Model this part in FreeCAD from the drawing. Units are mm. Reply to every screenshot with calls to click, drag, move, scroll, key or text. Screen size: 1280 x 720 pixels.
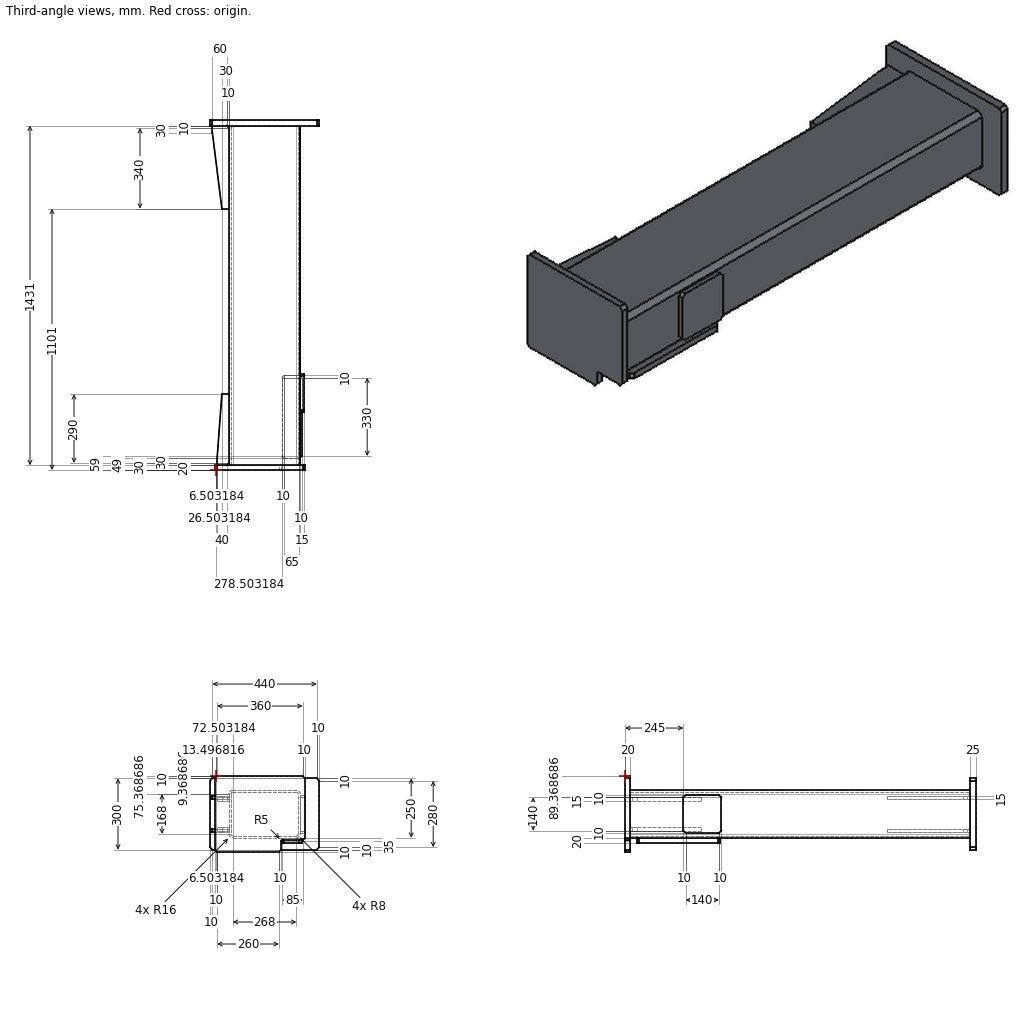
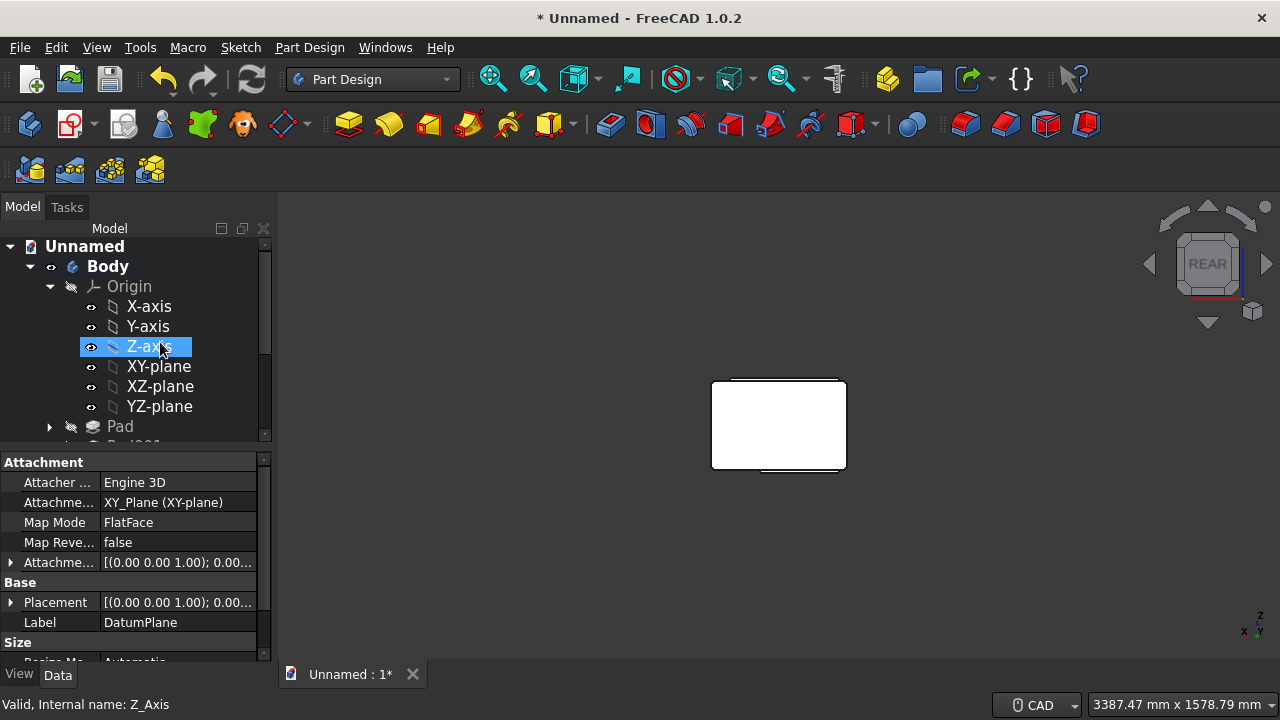
click(136, 367)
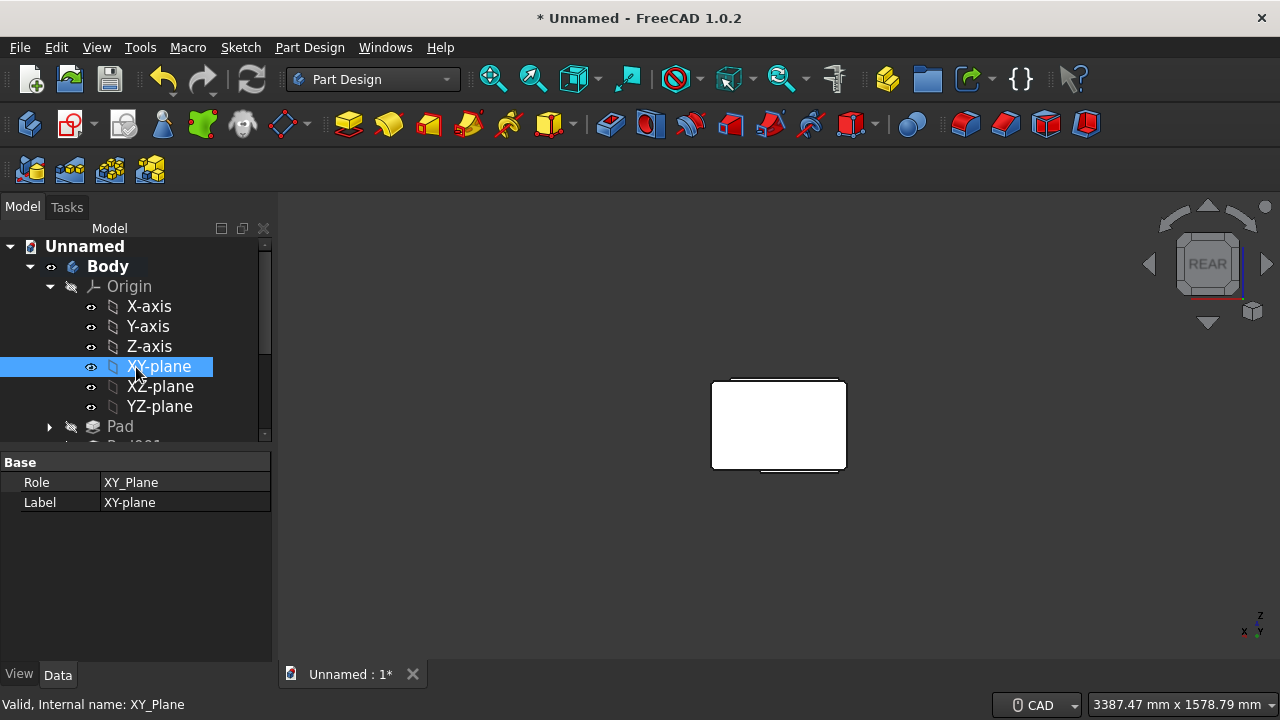
click(284, 124)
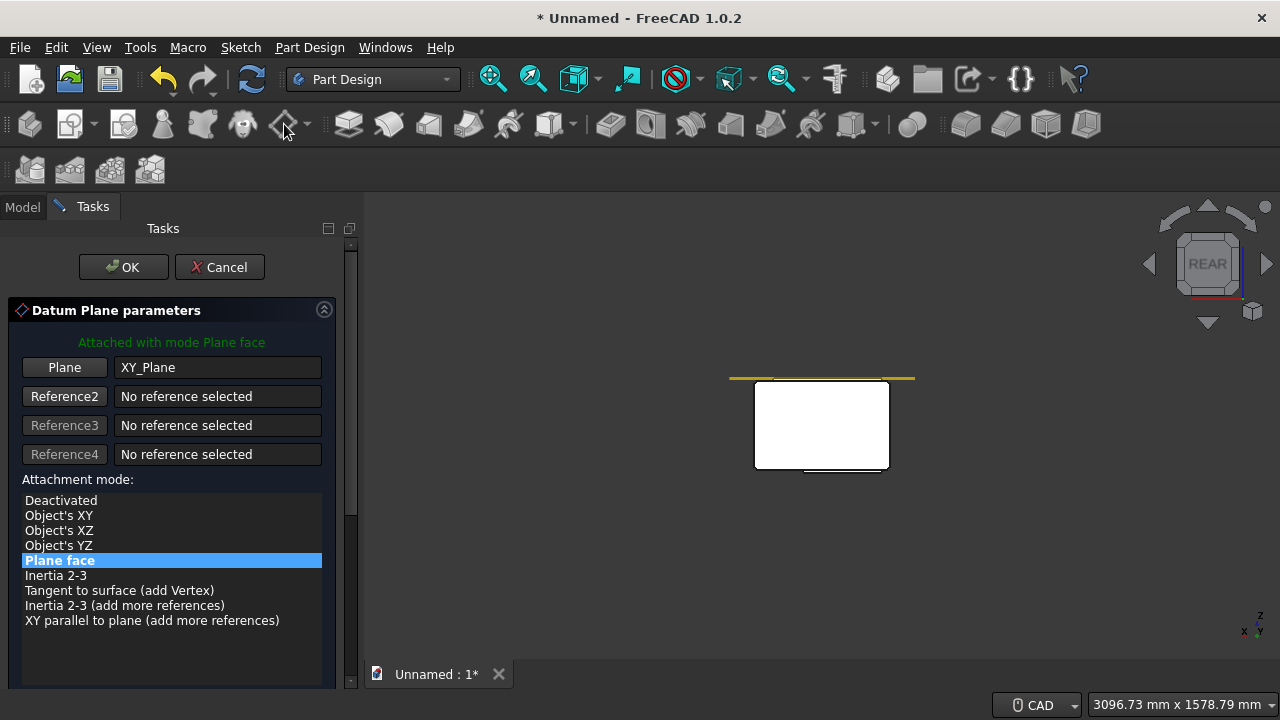
scroll(351, 463, down, 3)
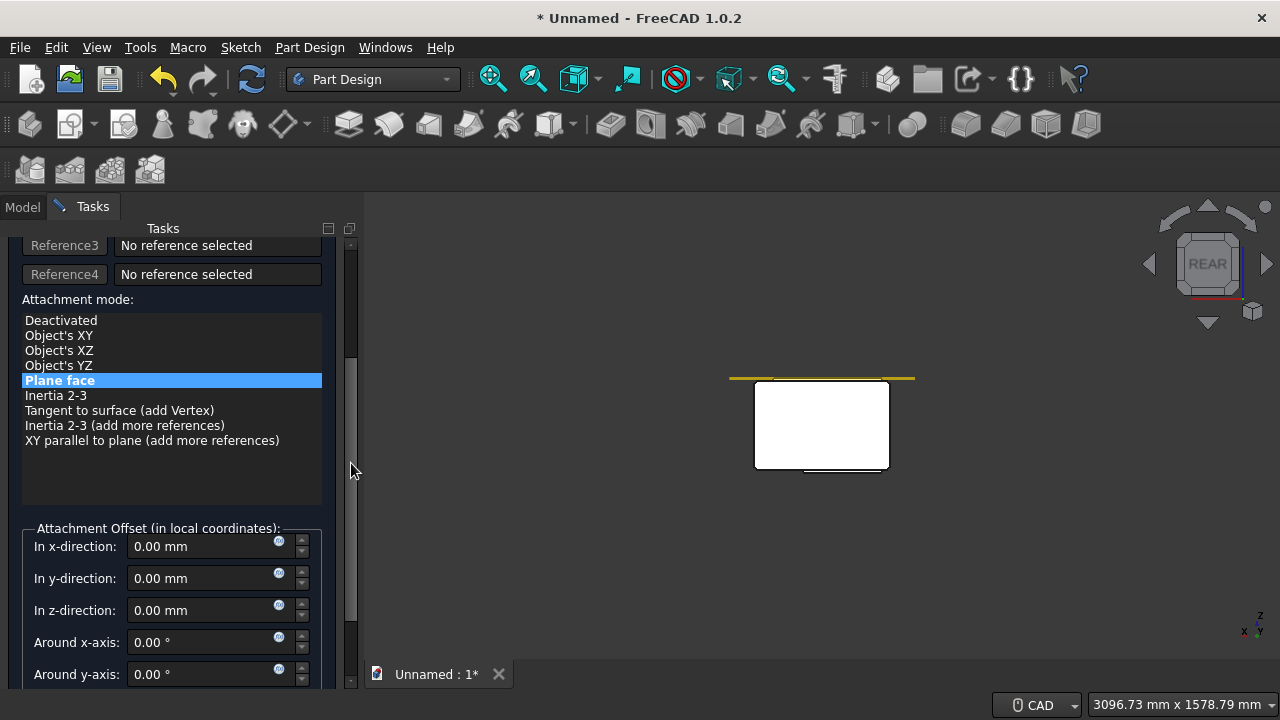
triple_click(210, 610)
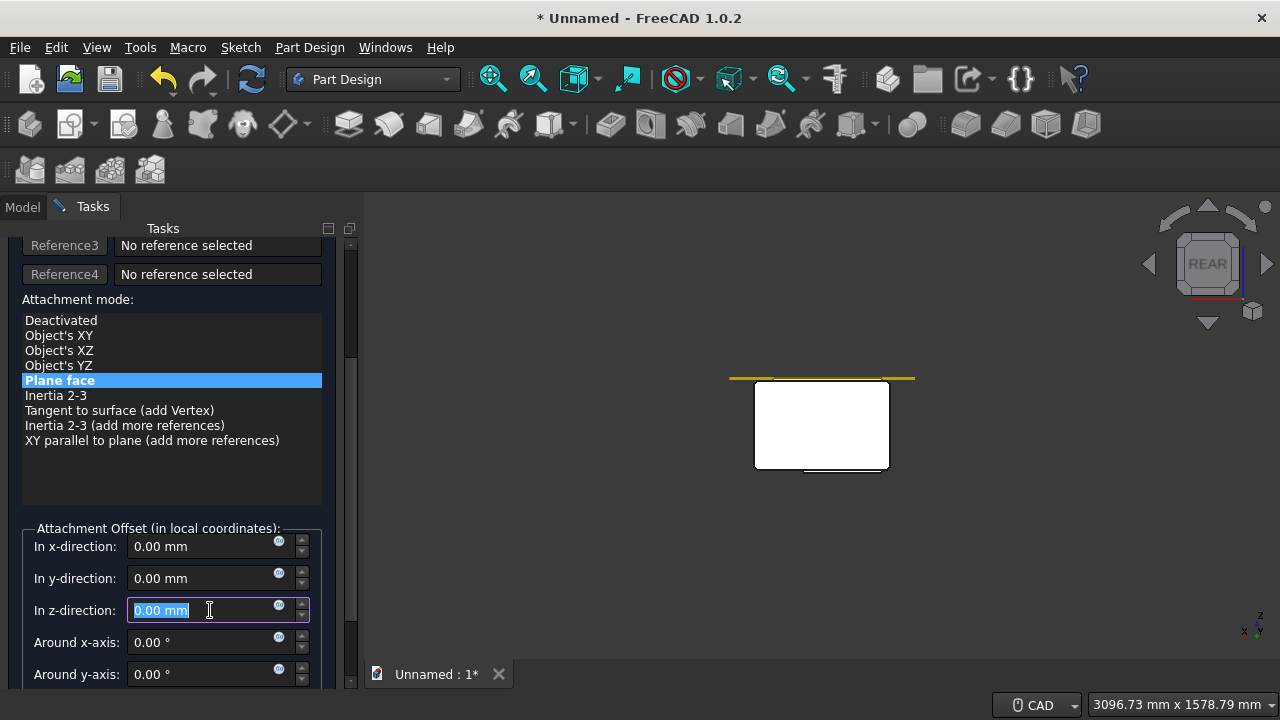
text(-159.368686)
key(Tab)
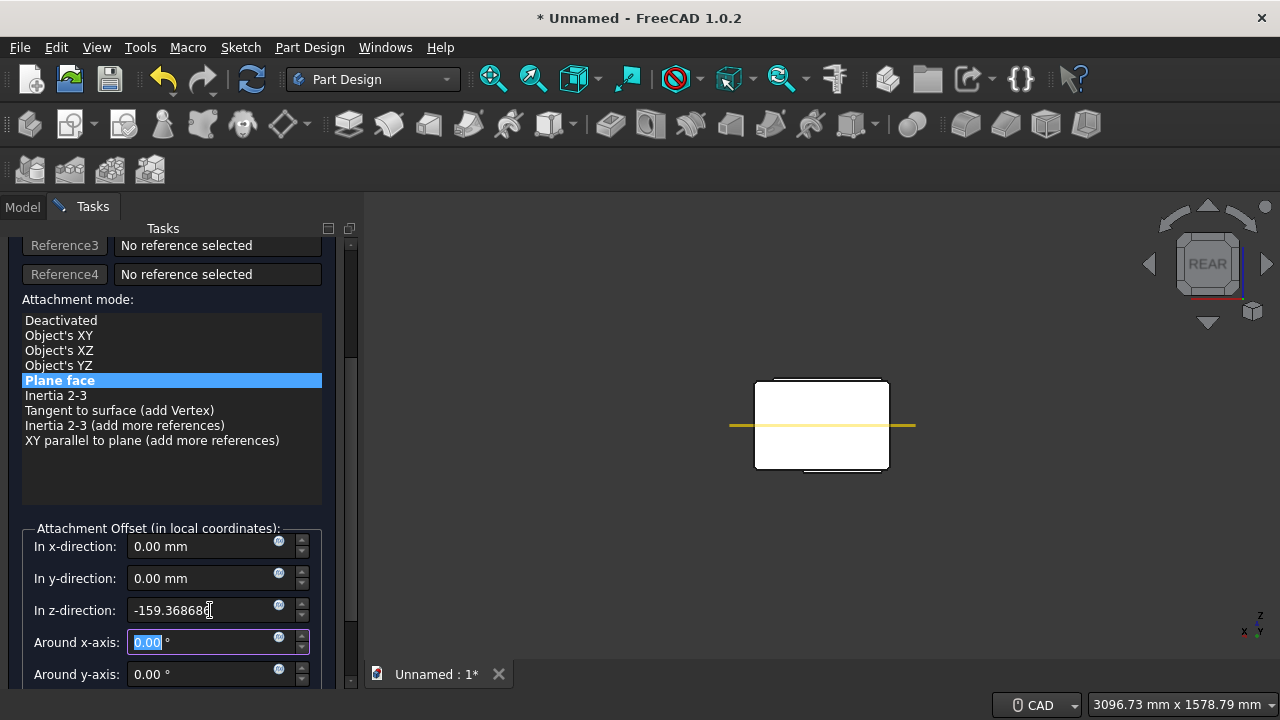
scroll(351, 463, up, 4)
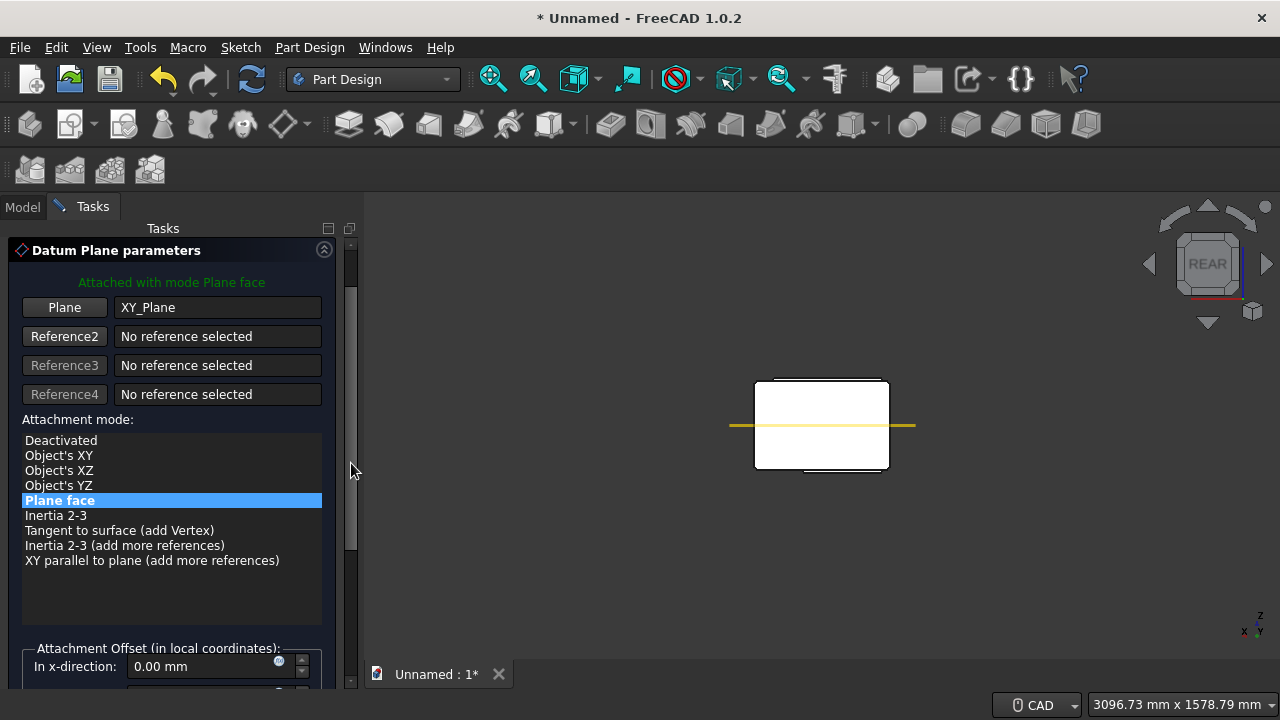
click(124, 267)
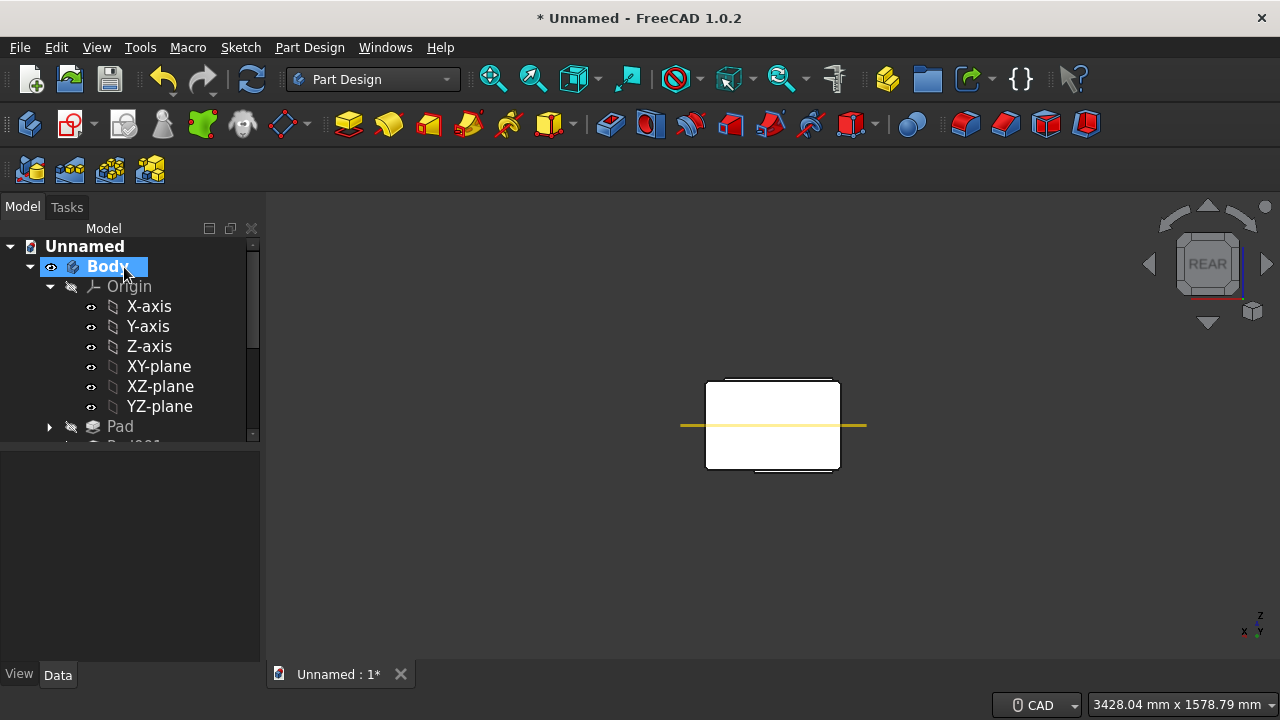
scroll(100, 342, down, 3)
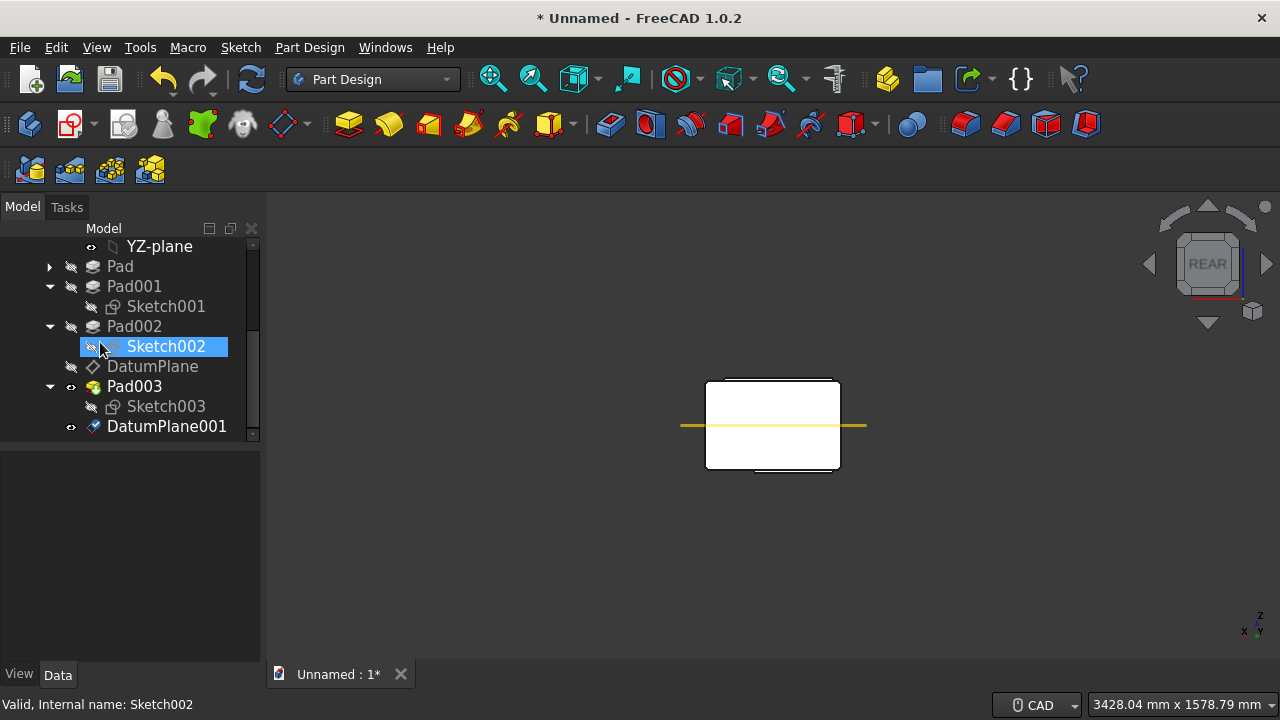
click(116, 387)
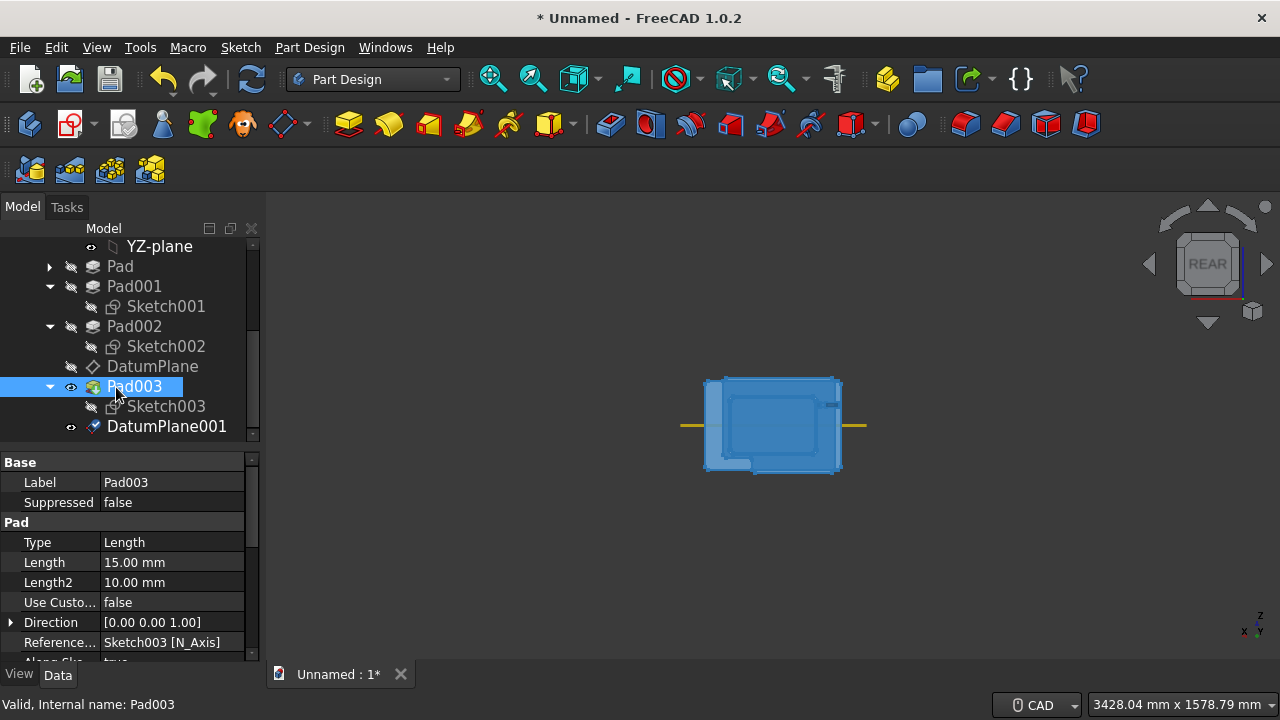
click(30, 170)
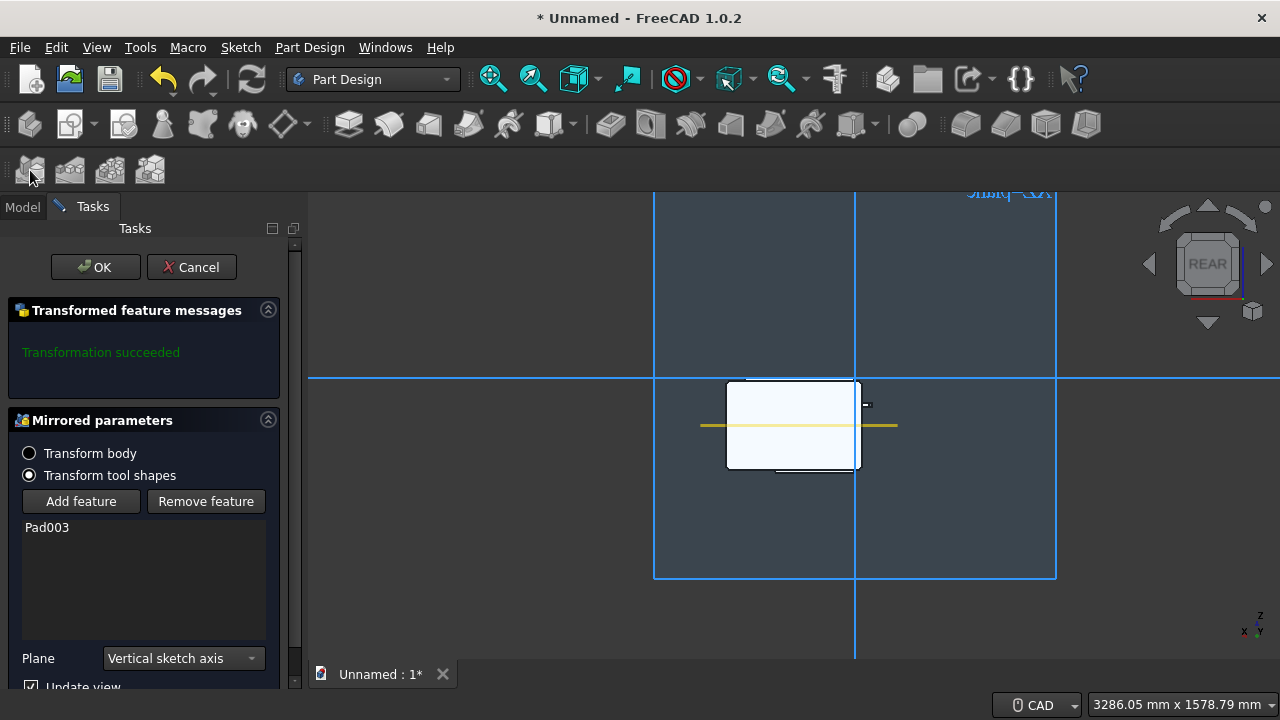
click(184, 658)